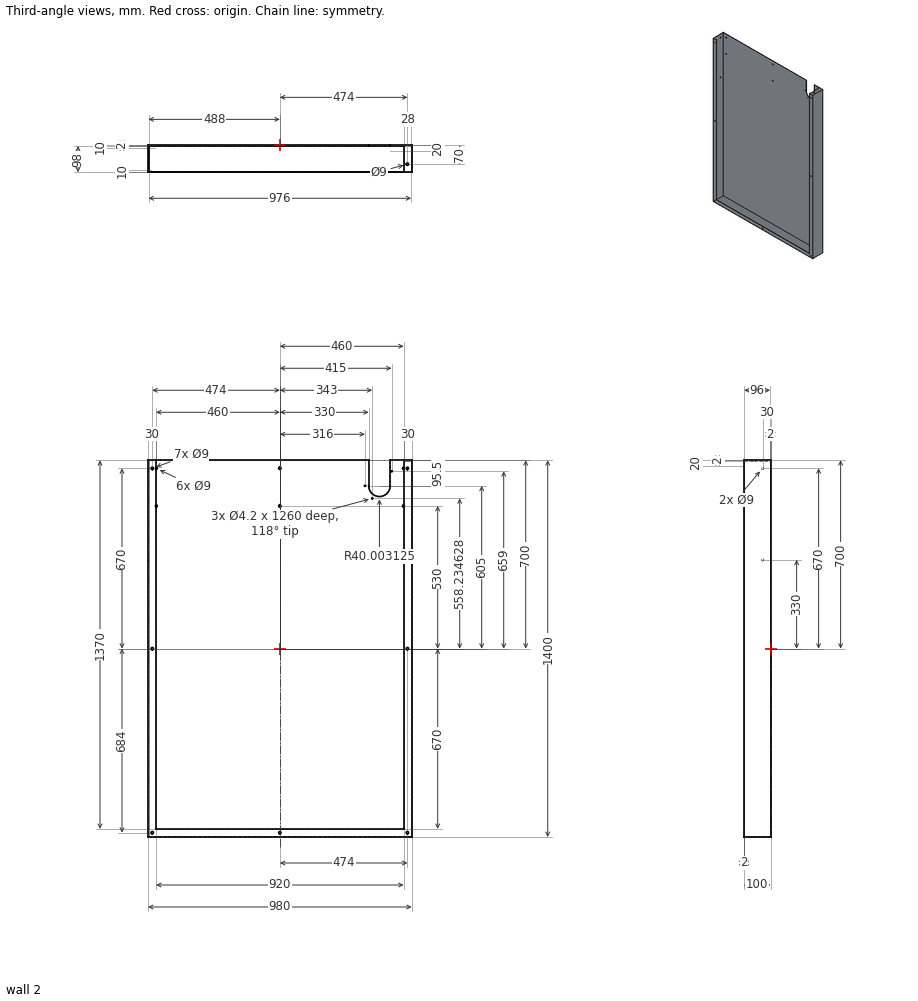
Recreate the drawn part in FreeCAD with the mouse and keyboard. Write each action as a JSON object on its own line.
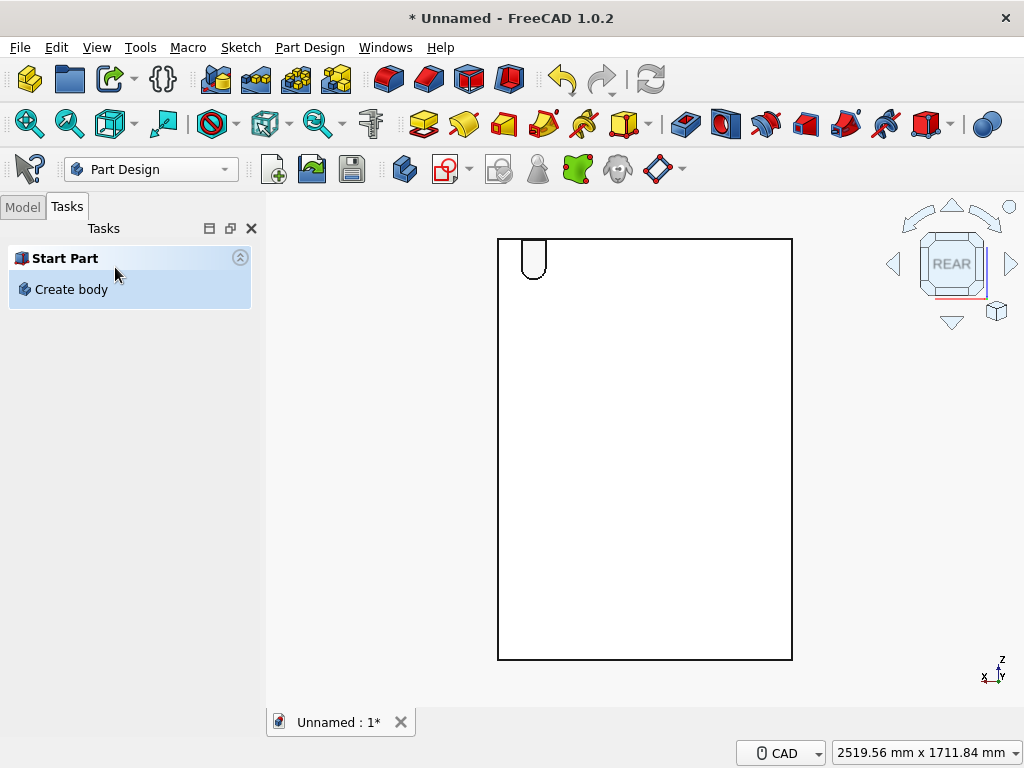
{"action": "key", "text": "0"}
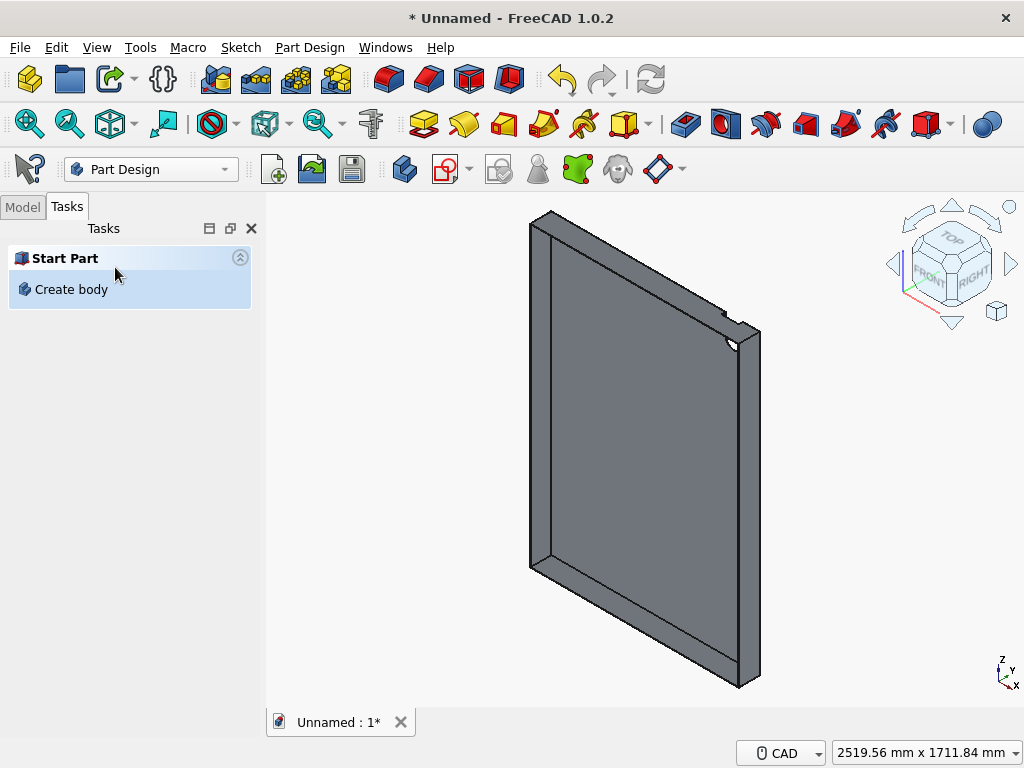
{"action": "left_click", "coordinate": [705, 311]}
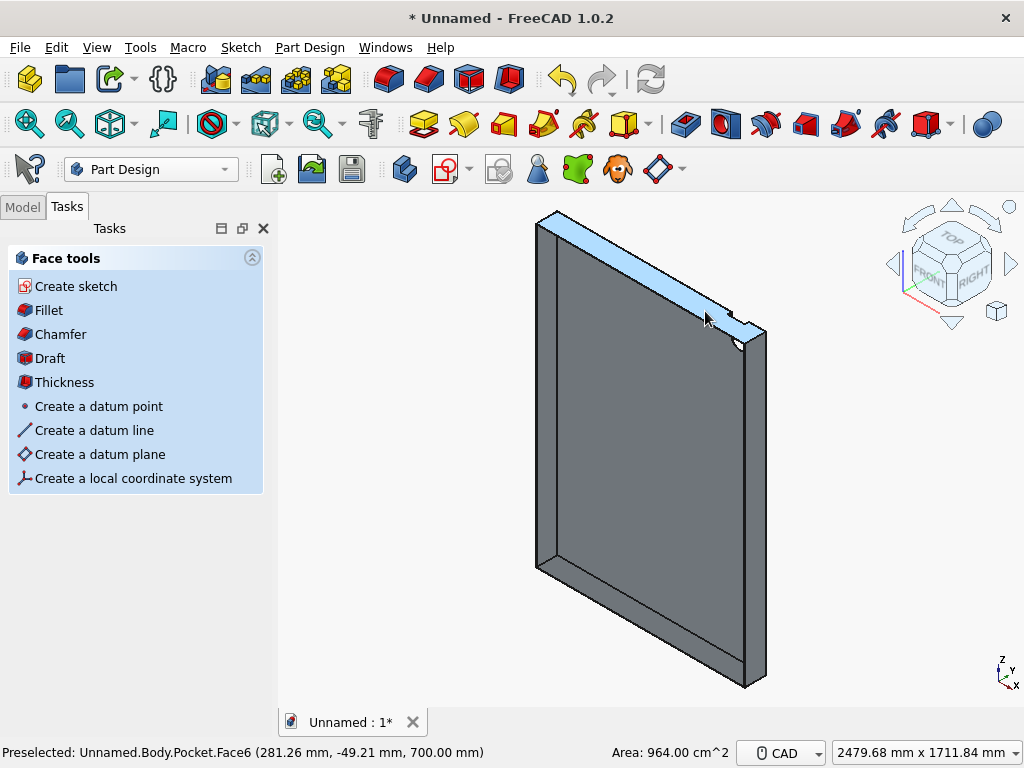
{"action": "left_click", "coordinate": [446, 170]}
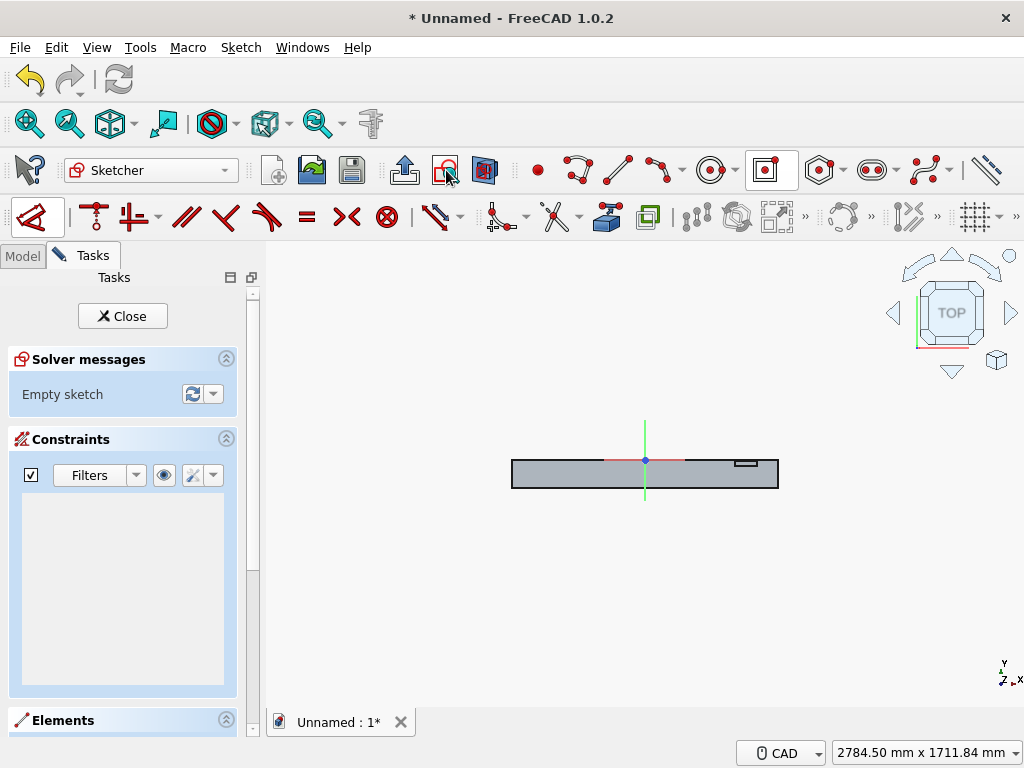
{"action": "scroll", "coordinate": [784, 474], "scroll_direction": "up", "scroll_amount": 2}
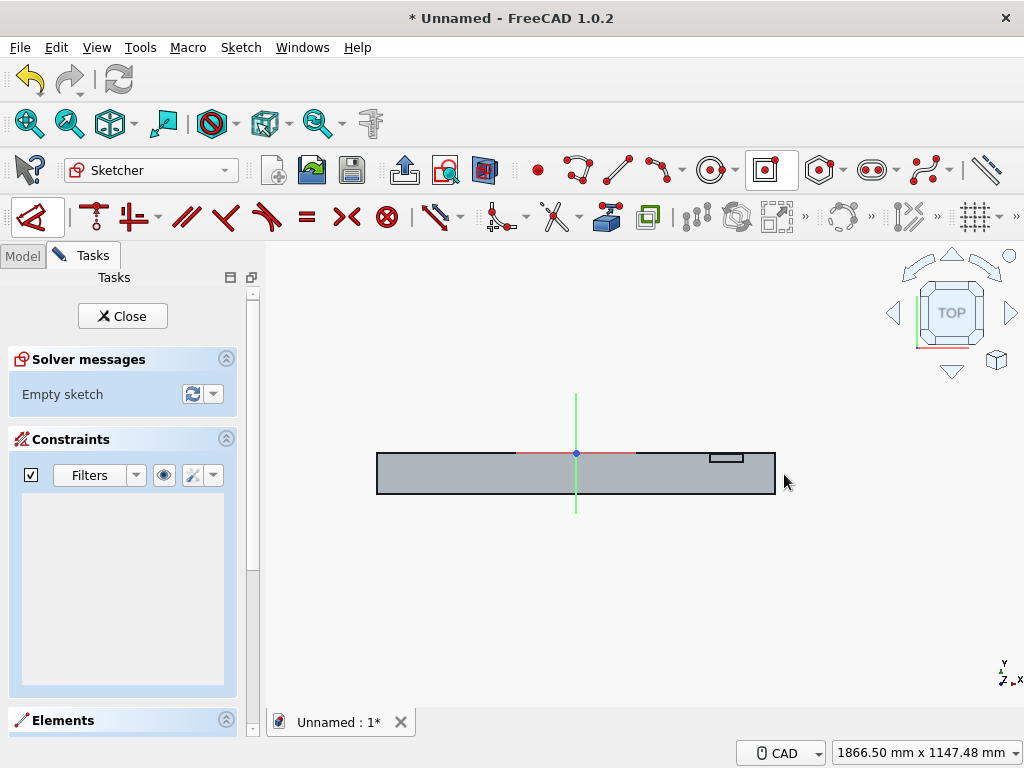
{"action": "left_click", "coordinate": [792, 170]}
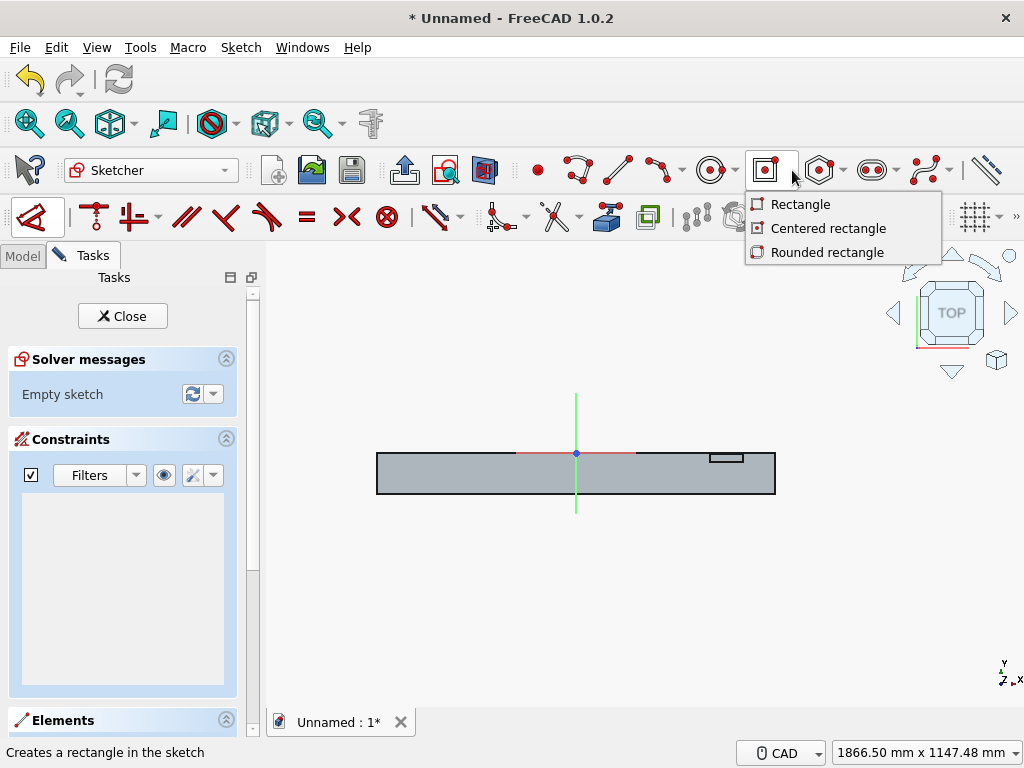
{"action": "left_click", "coordinate": [844, 204]}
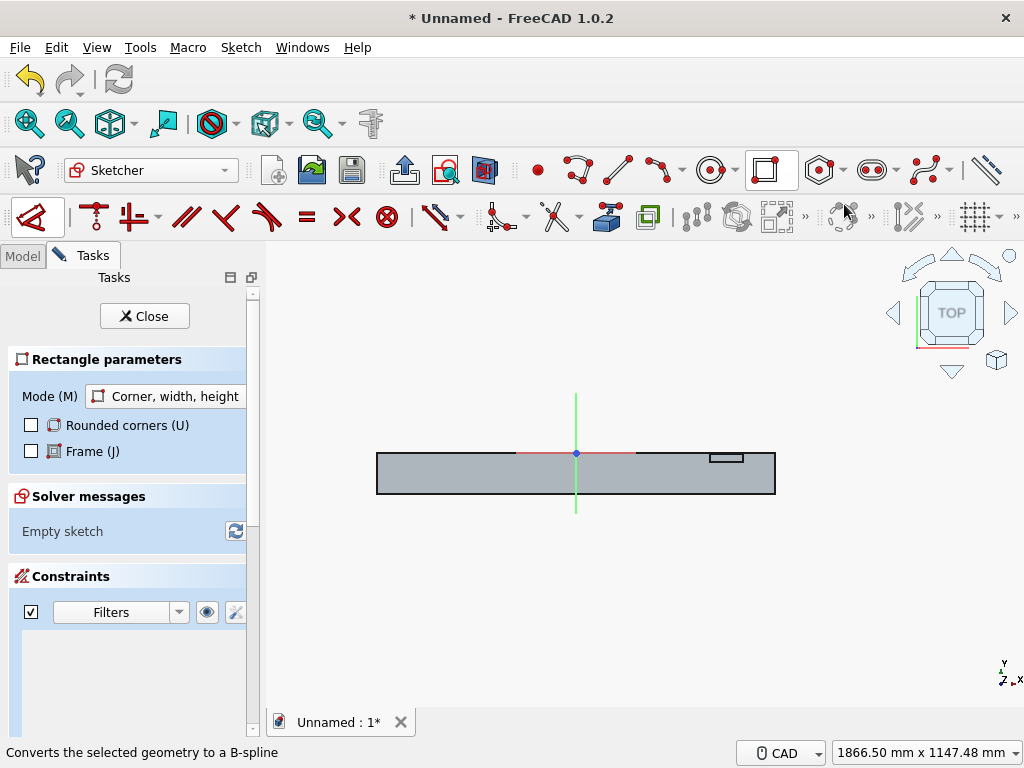
{"action": "scroll", "coordinate": [378, 454], "scroll_direction": "up", "scroll_amount": 15}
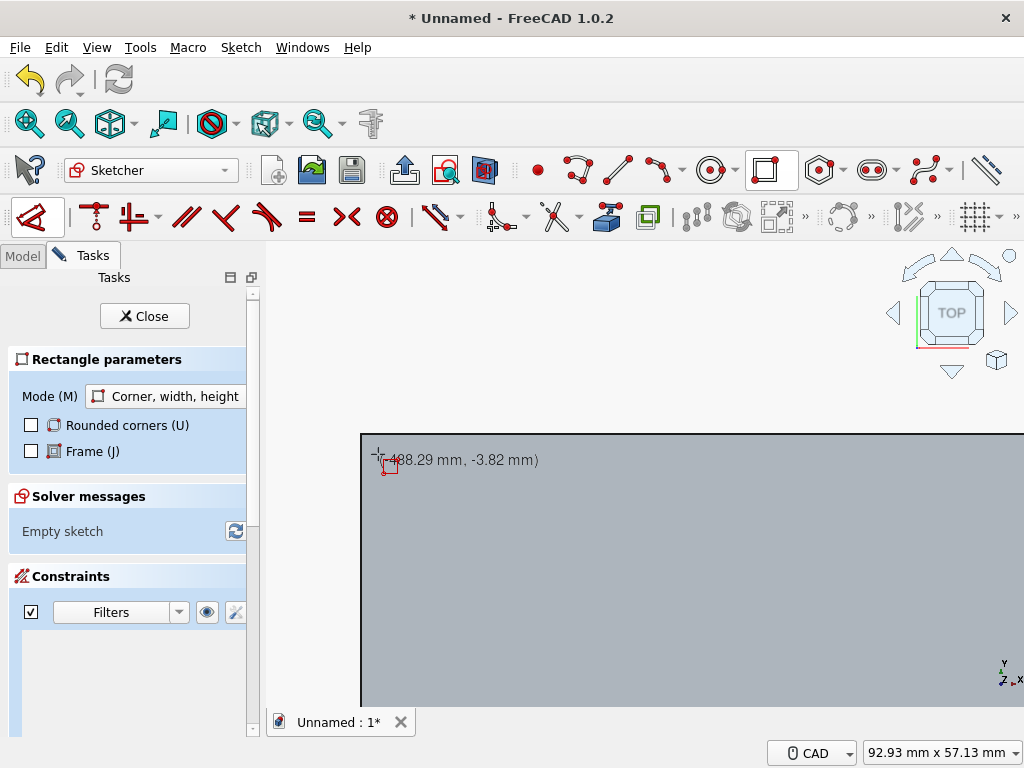
{"action": "left_click", "coordinate": [378, 450]}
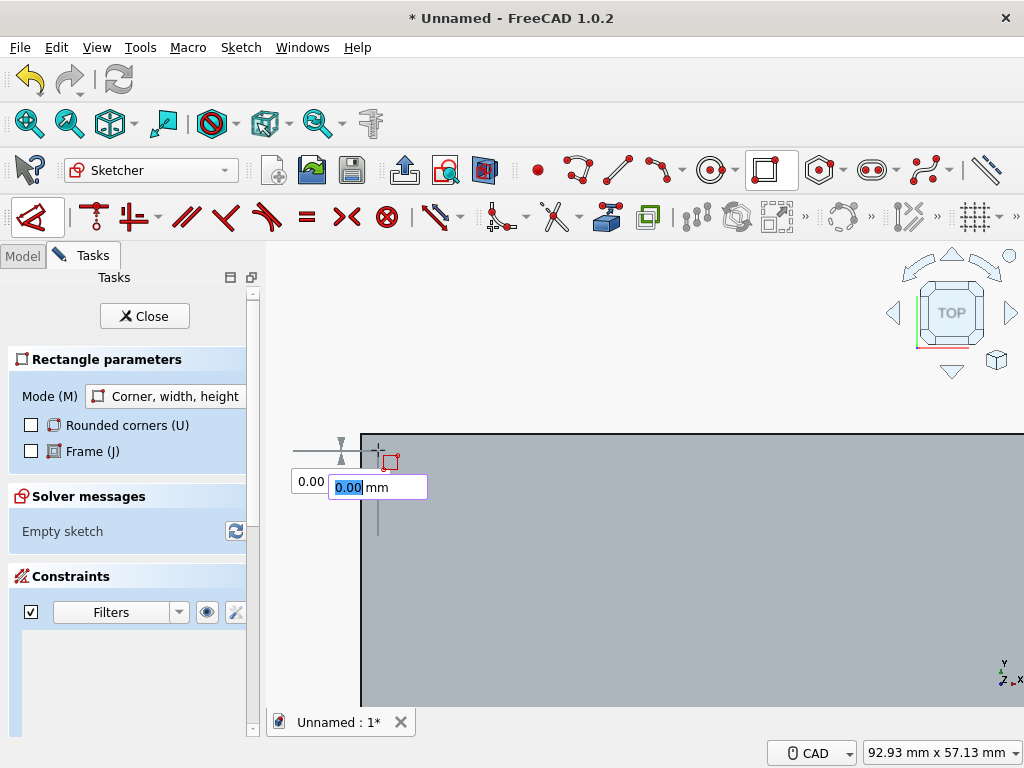
{"action": "scroll", "coordinate": [378, 455], "scroll_direction": "down", "scroll_amount": 15}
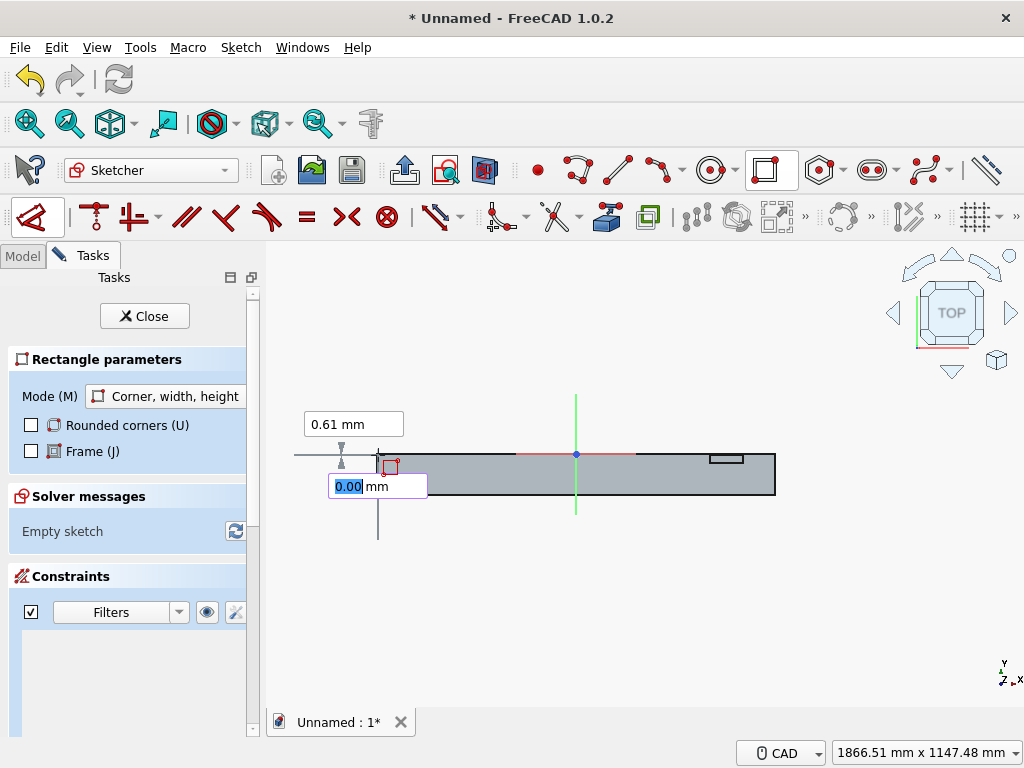
{"action": "left_click", "coordinate": [774, 495]}
{"action": "key", "text": "Escape"}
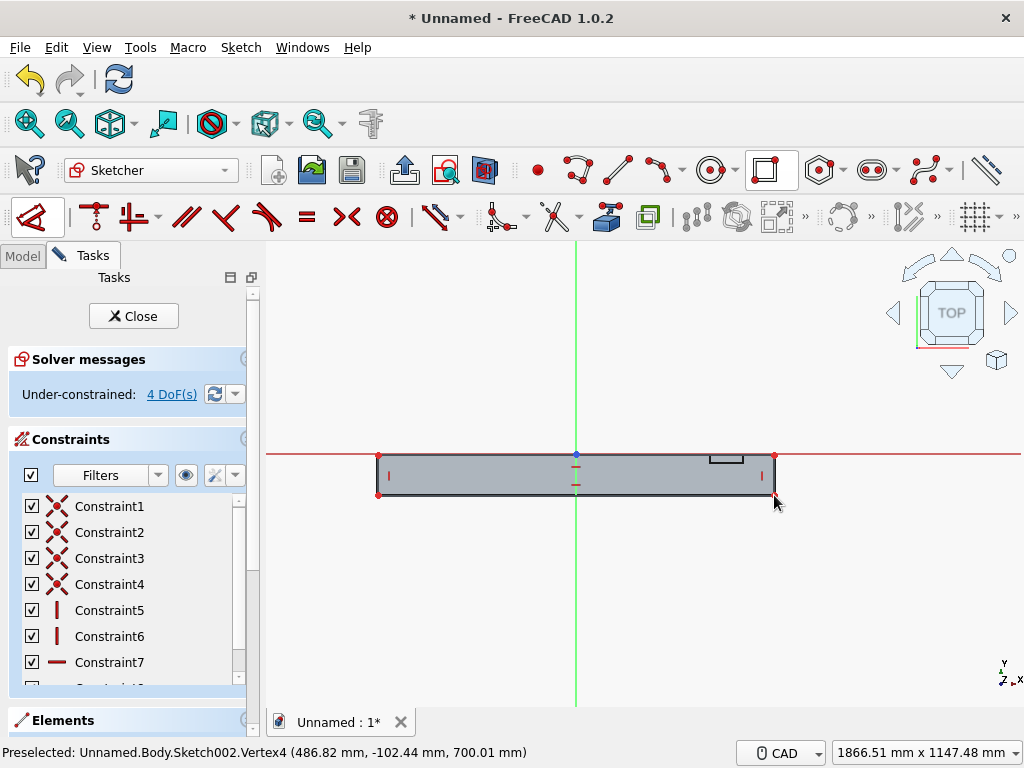
{"action": "left_click", "coordinate": [378, 467]}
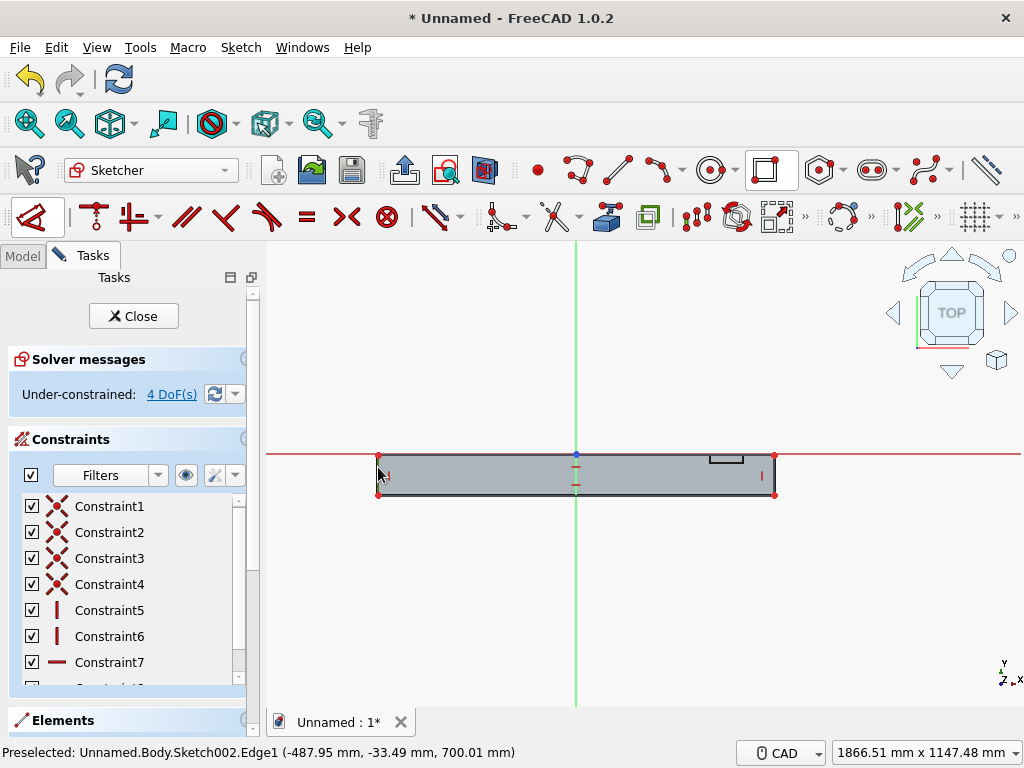
{"action": "left_click", "coordinate": [58, 218]}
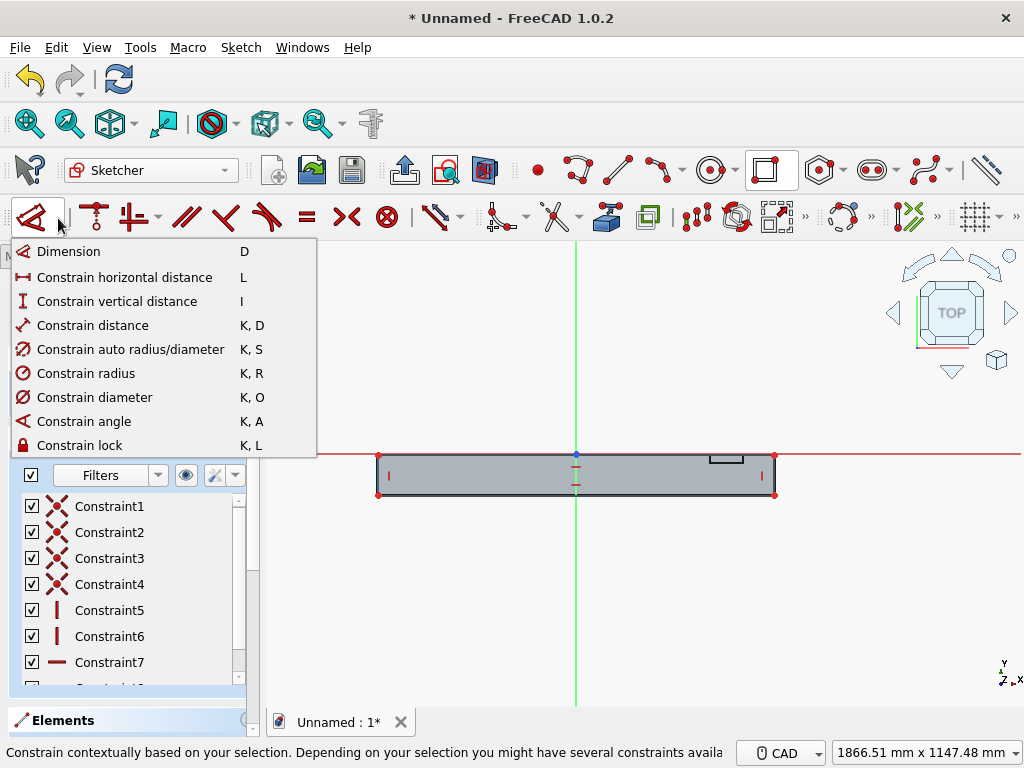
{"action": "left_click", "coordinate": [164, 301]}